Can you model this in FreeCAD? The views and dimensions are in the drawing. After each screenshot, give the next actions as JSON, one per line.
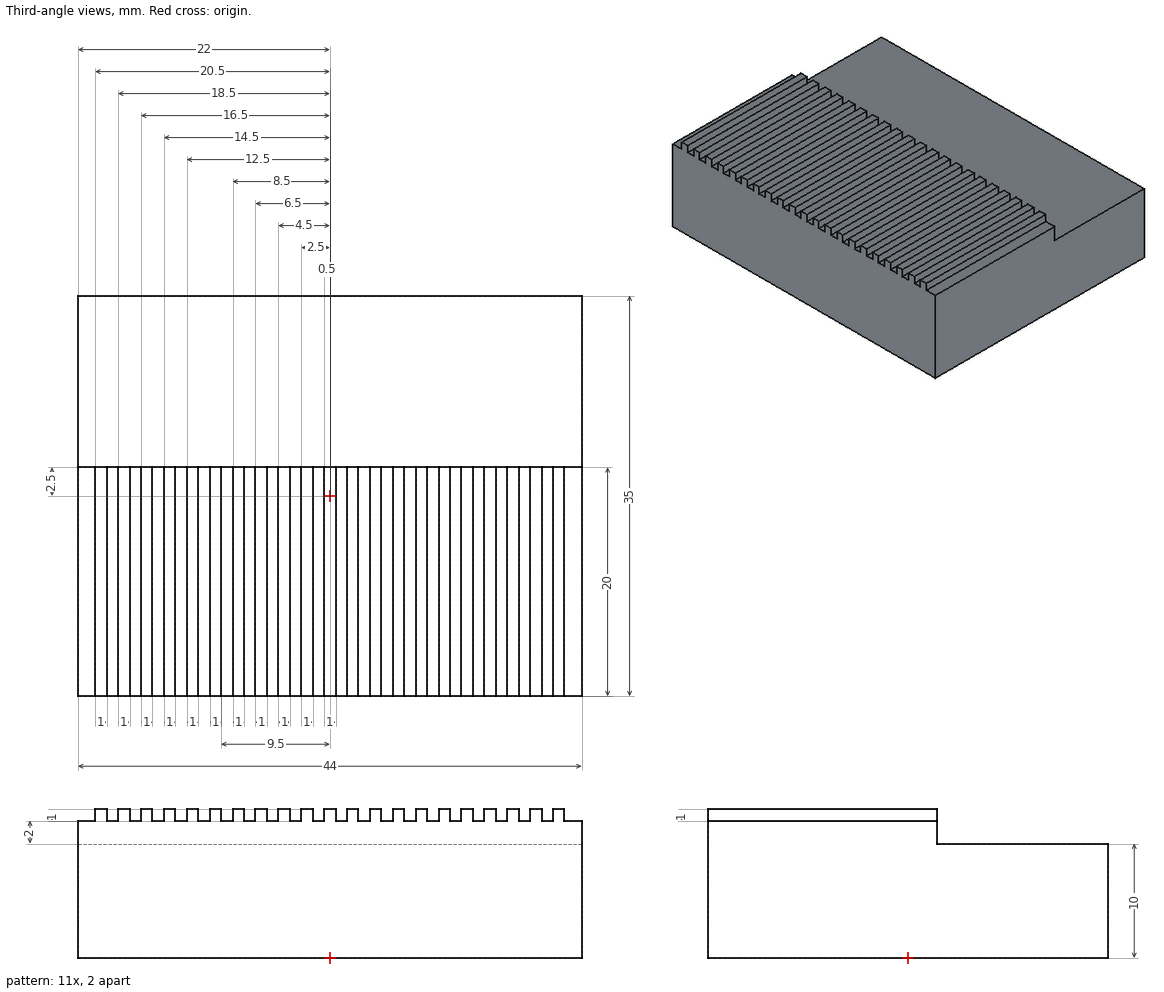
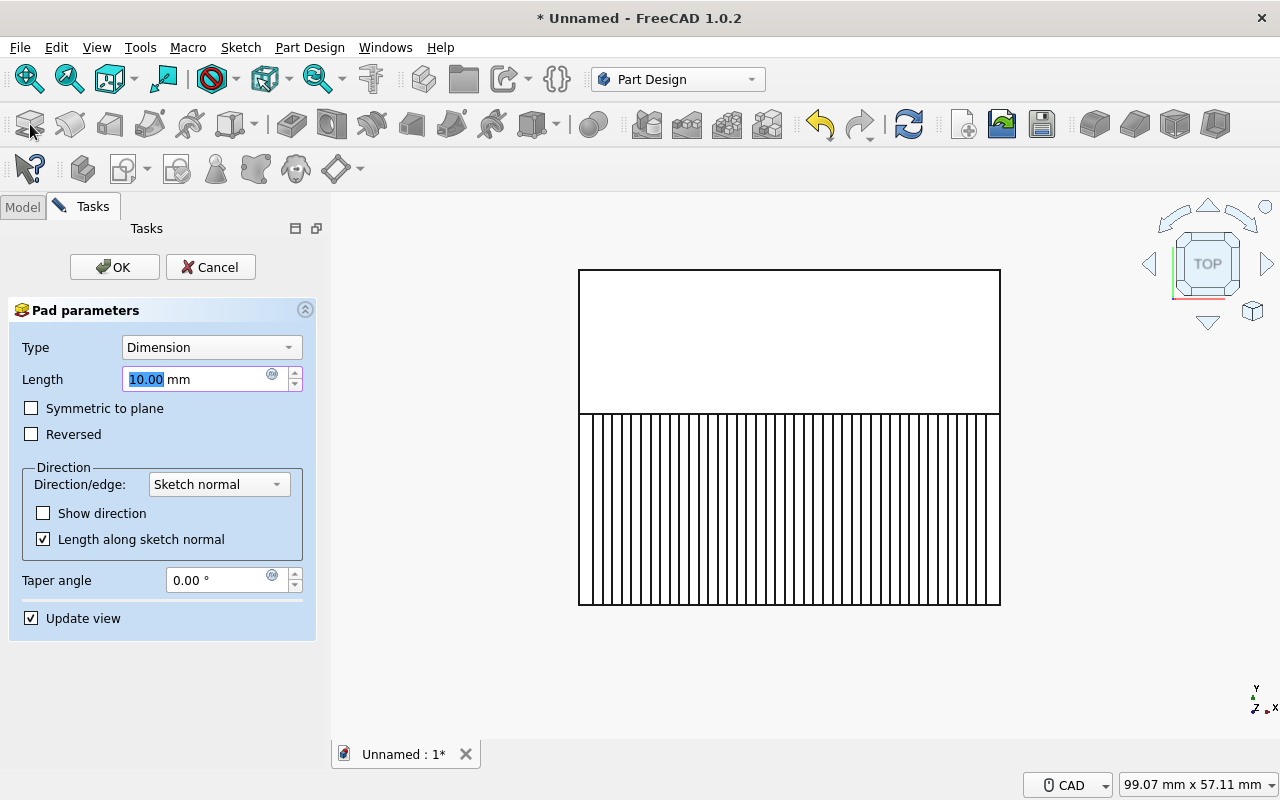
{"action": "type", "text": "1"}
{"action": "key", "text": "Tab"}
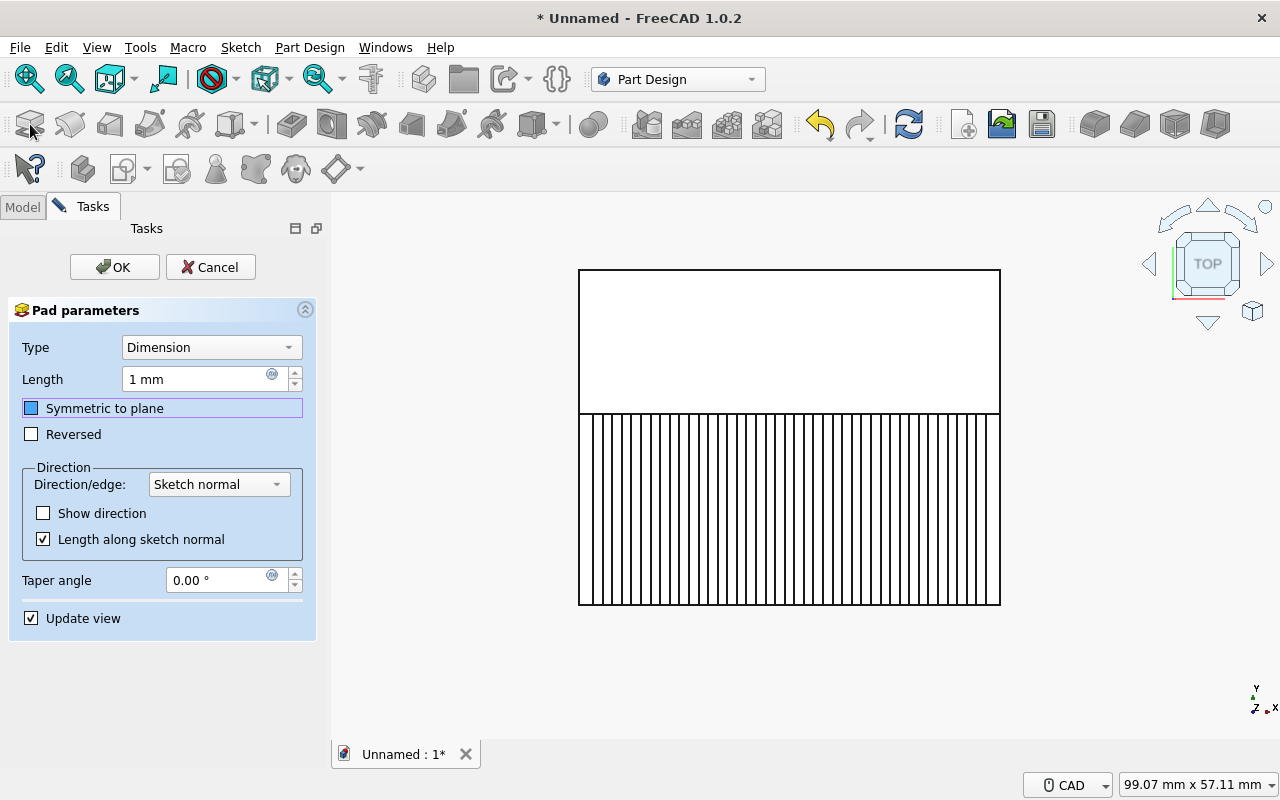
{"action": "left_click", "coordinate": [115, 267]}